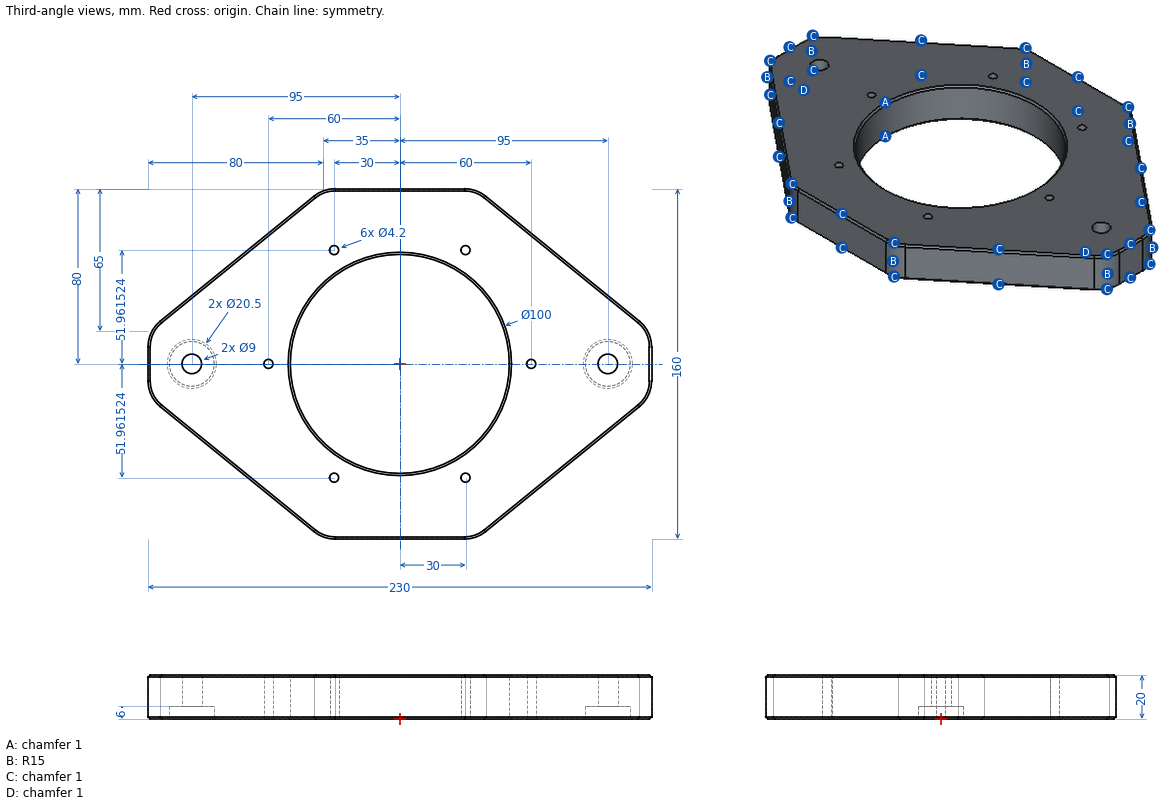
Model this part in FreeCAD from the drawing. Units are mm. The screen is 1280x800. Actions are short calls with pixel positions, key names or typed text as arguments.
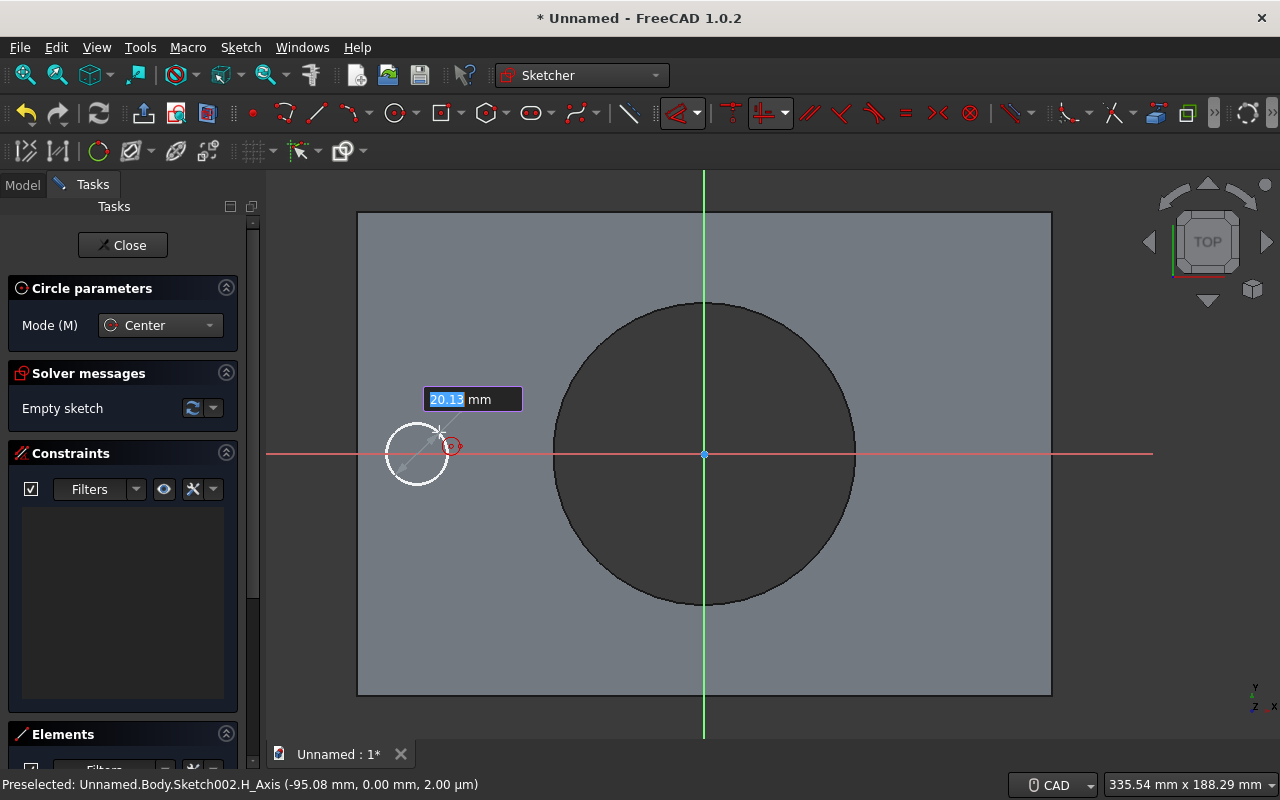
text(20.5)
key(Return)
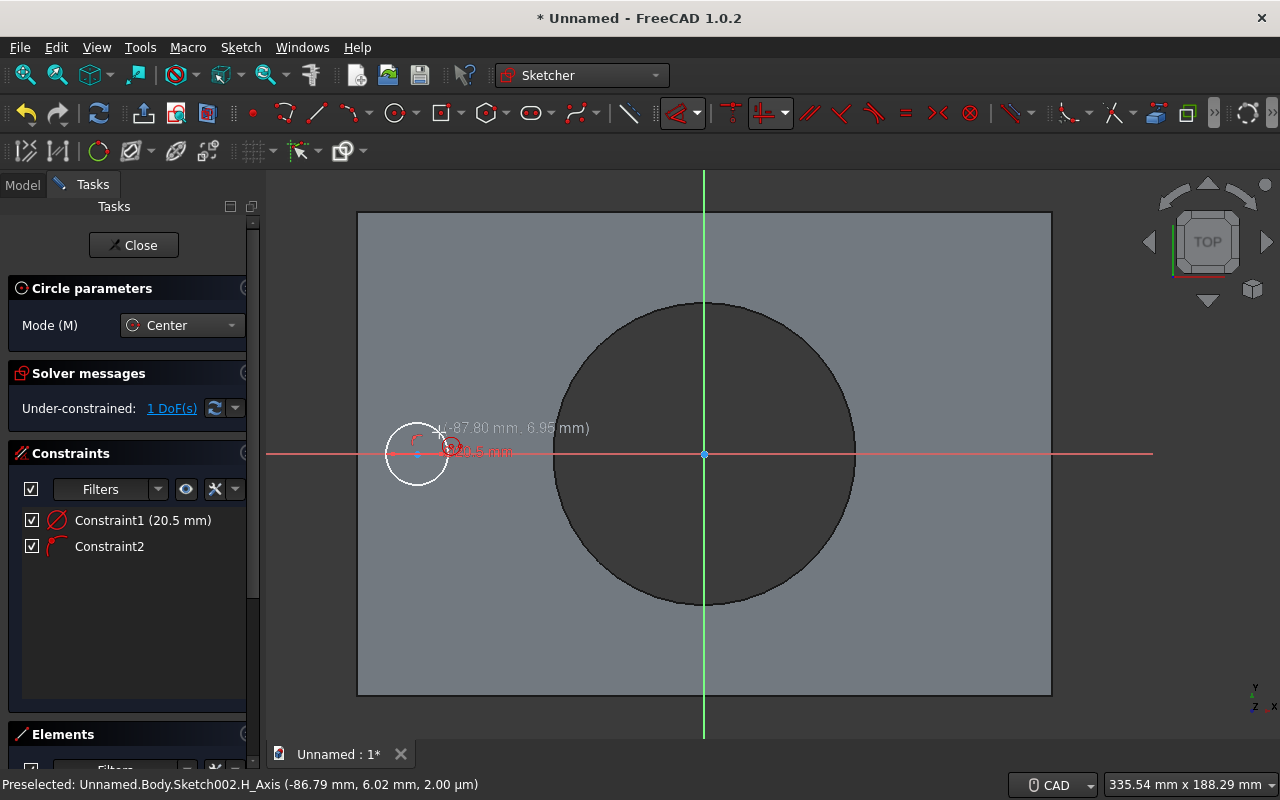
click(991, 454)
move(1013, 432)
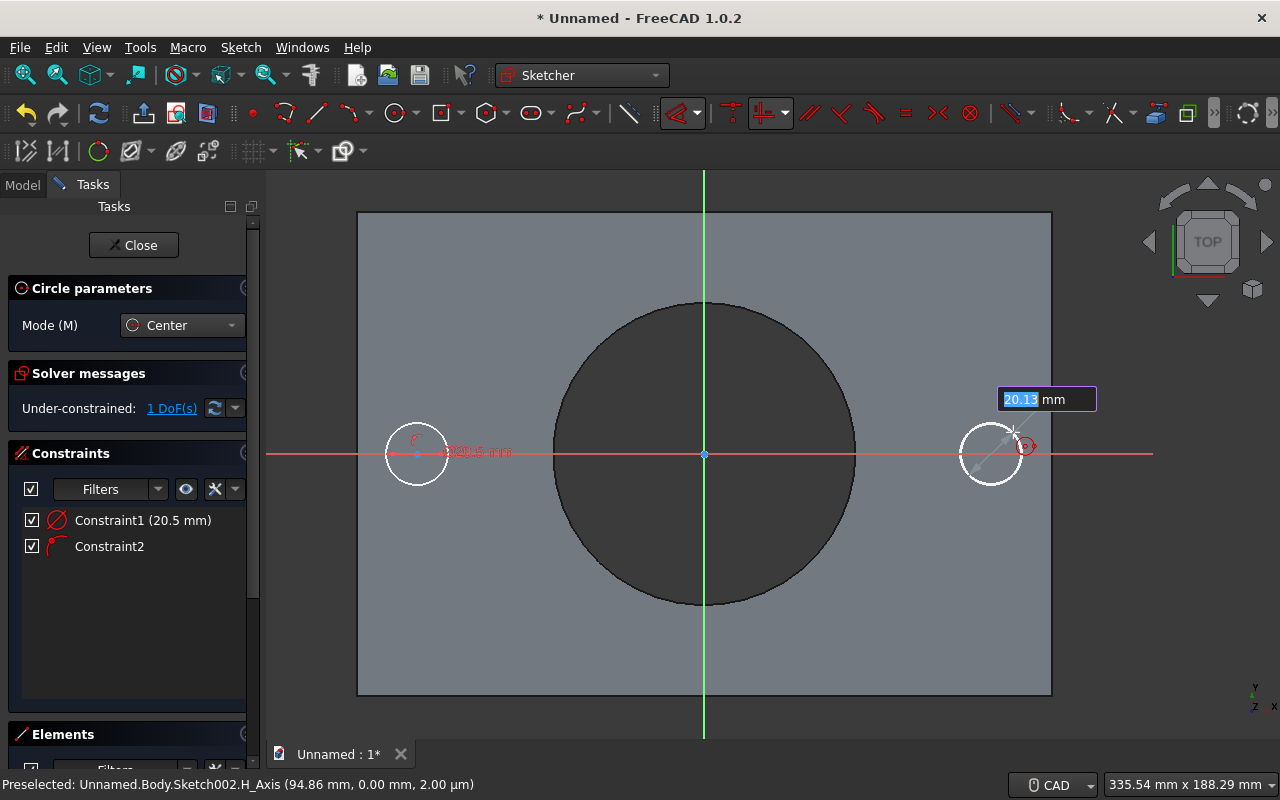
text(20.5)
key(Return)
key(Escape)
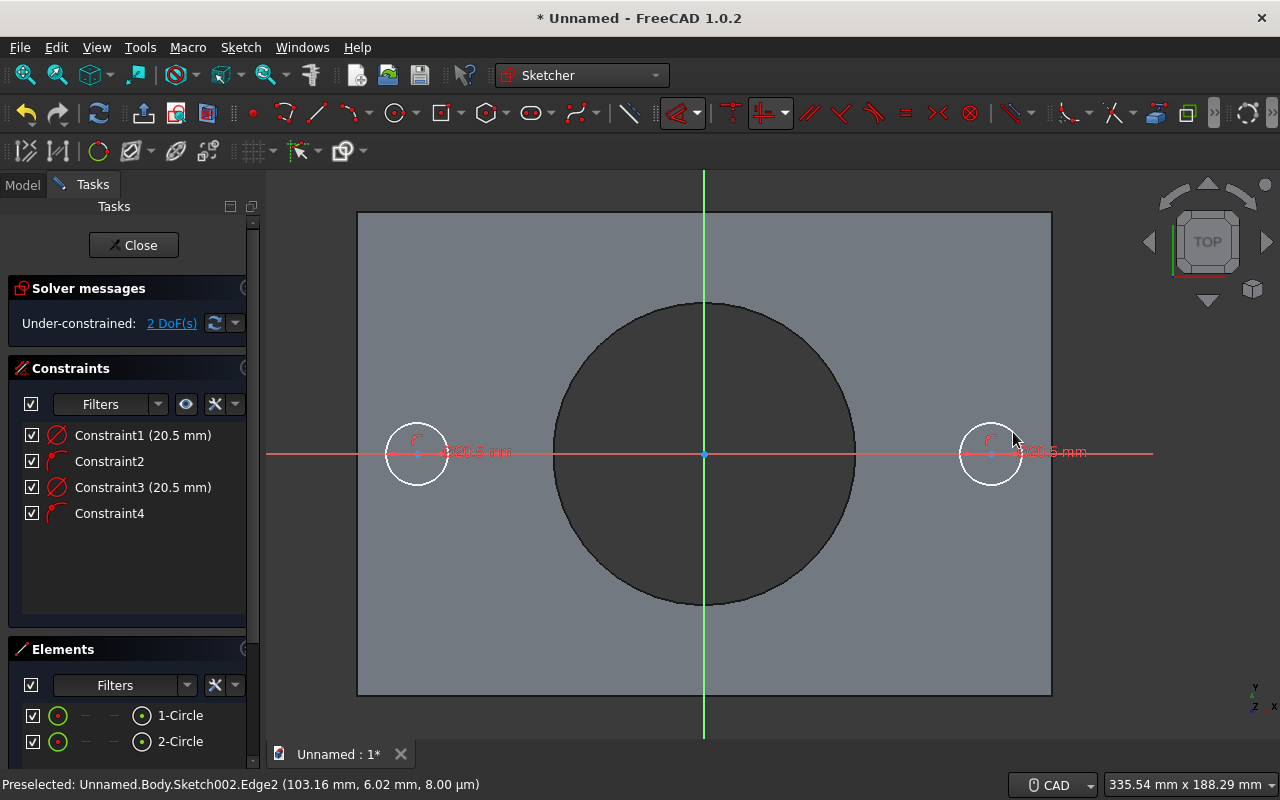
click(676, 114)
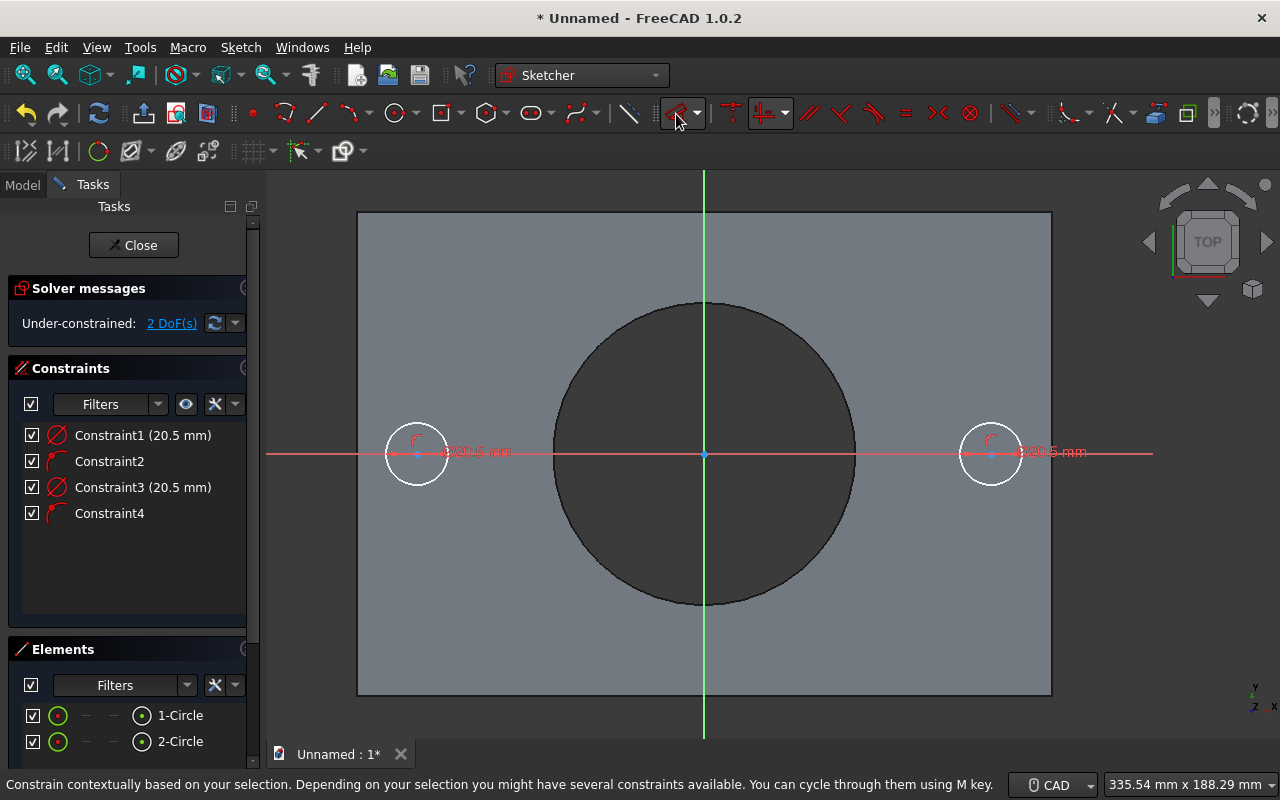
click(417, 454)
click(561, 488)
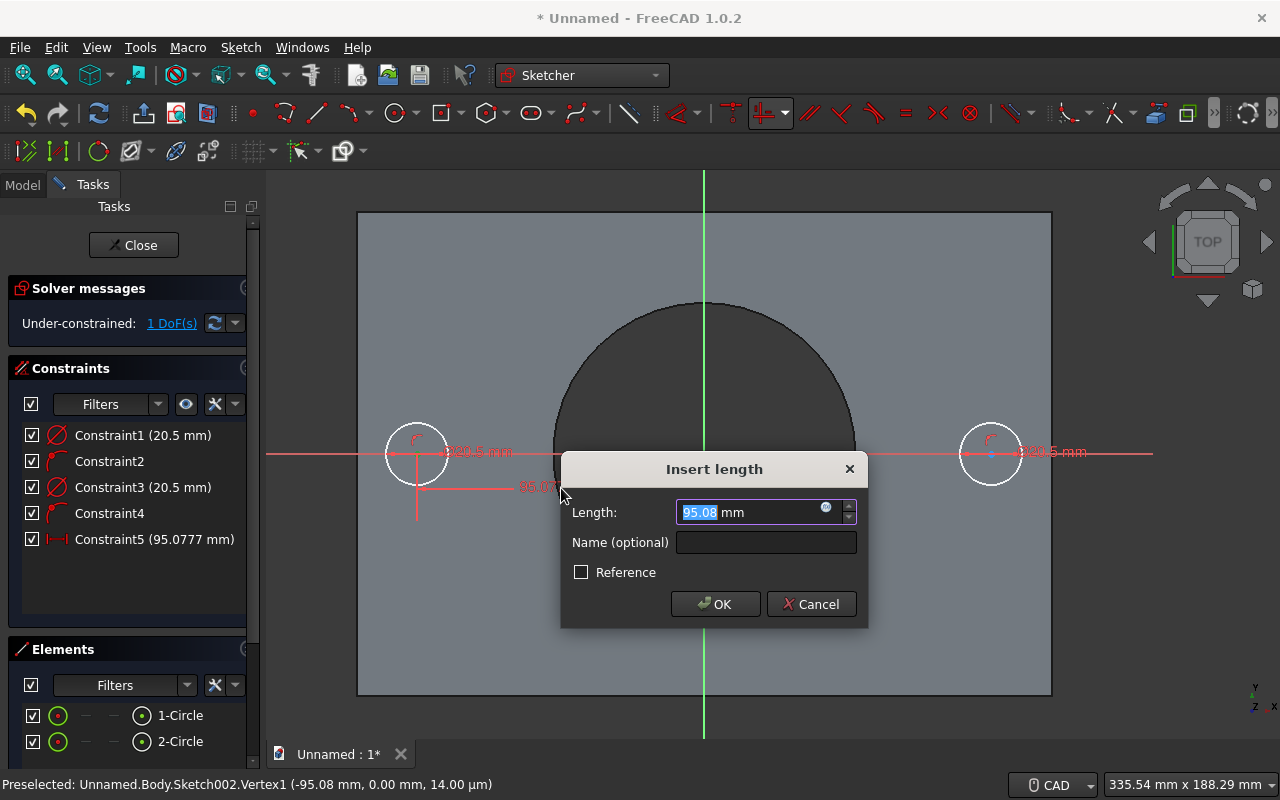
text(95)
key(Return)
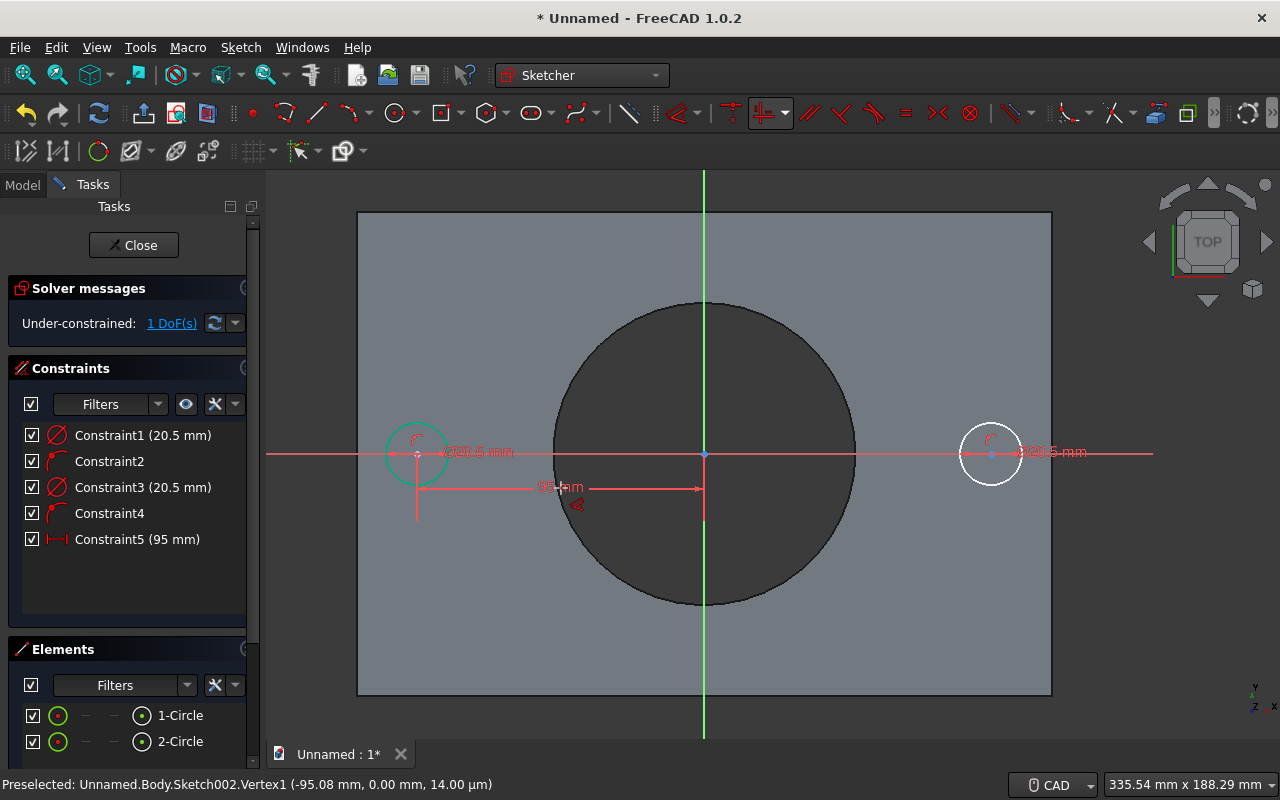
click(991, 454)
click(848, 488)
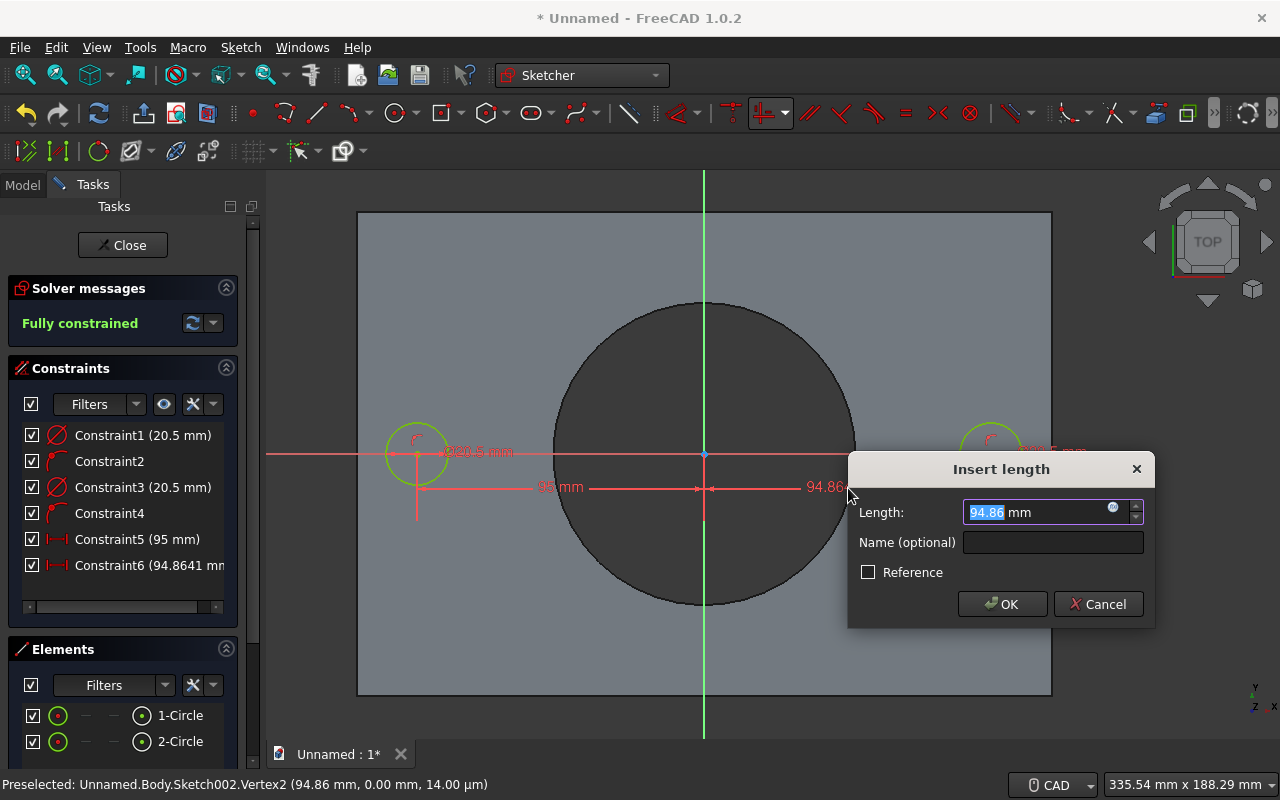
text(95)
key(Return)
key(Escape)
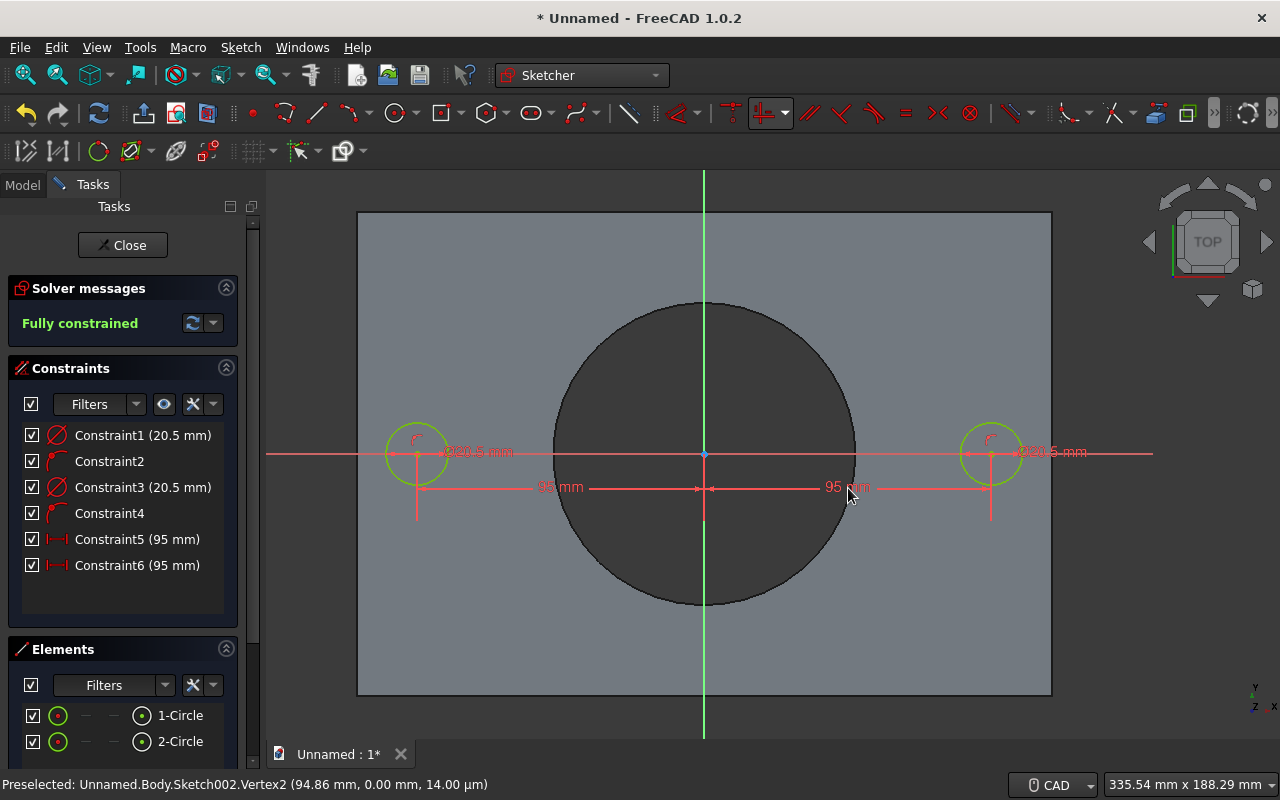
click(123, 245)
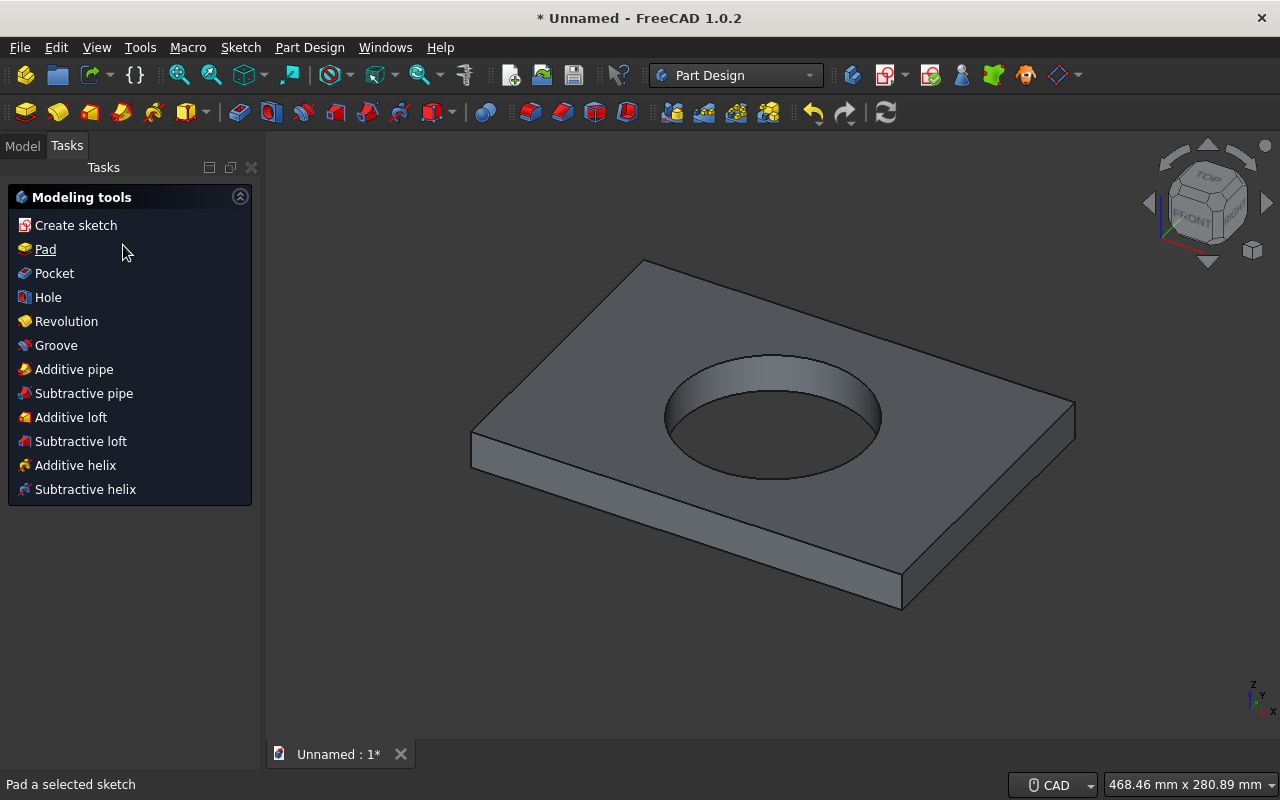
click(240, 112)